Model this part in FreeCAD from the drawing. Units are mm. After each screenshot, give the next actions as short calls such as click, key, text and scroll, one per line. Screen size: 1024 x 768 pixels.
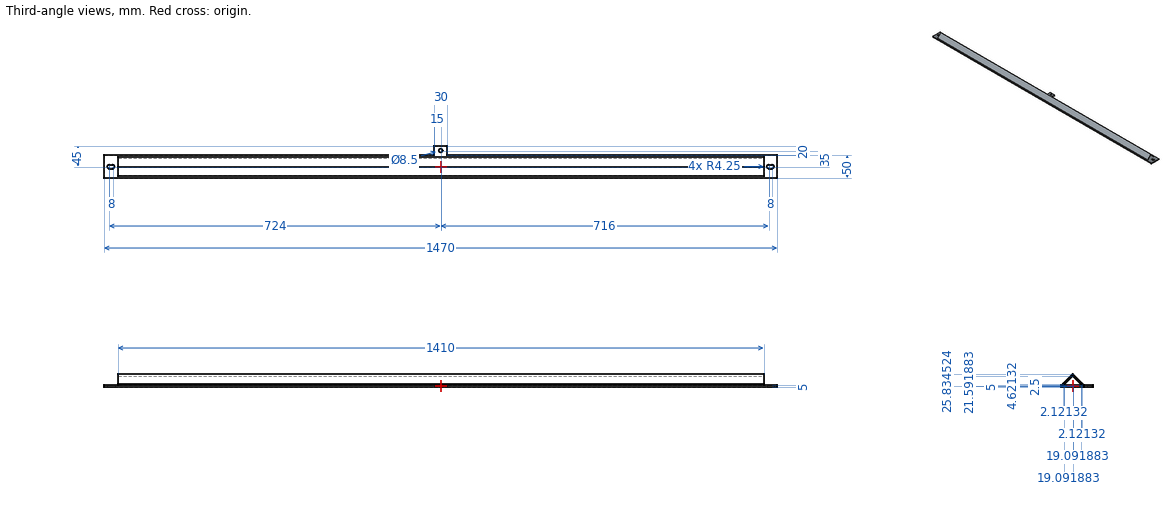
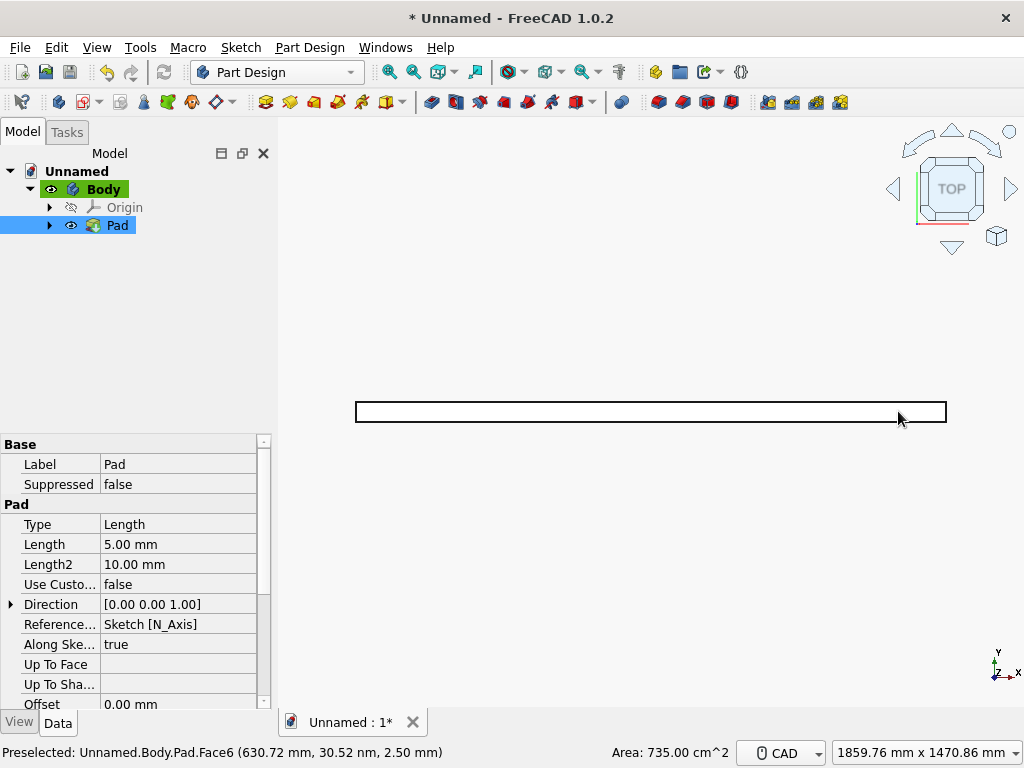
click(84, 102)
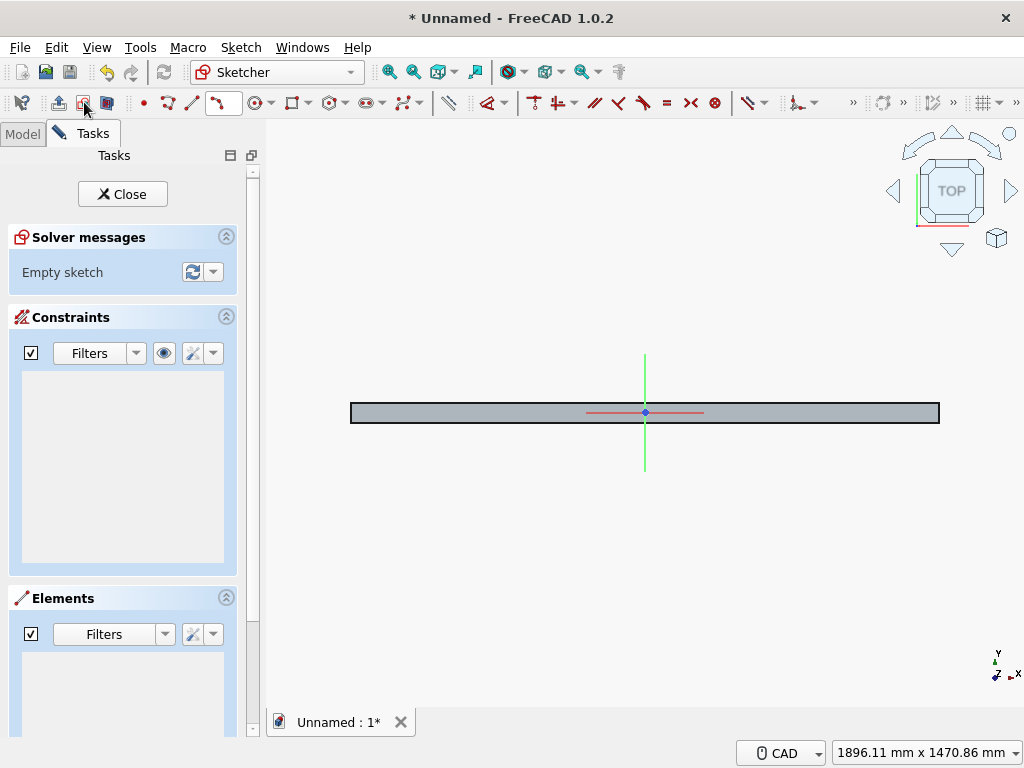
scroll(437, 413, down, 2)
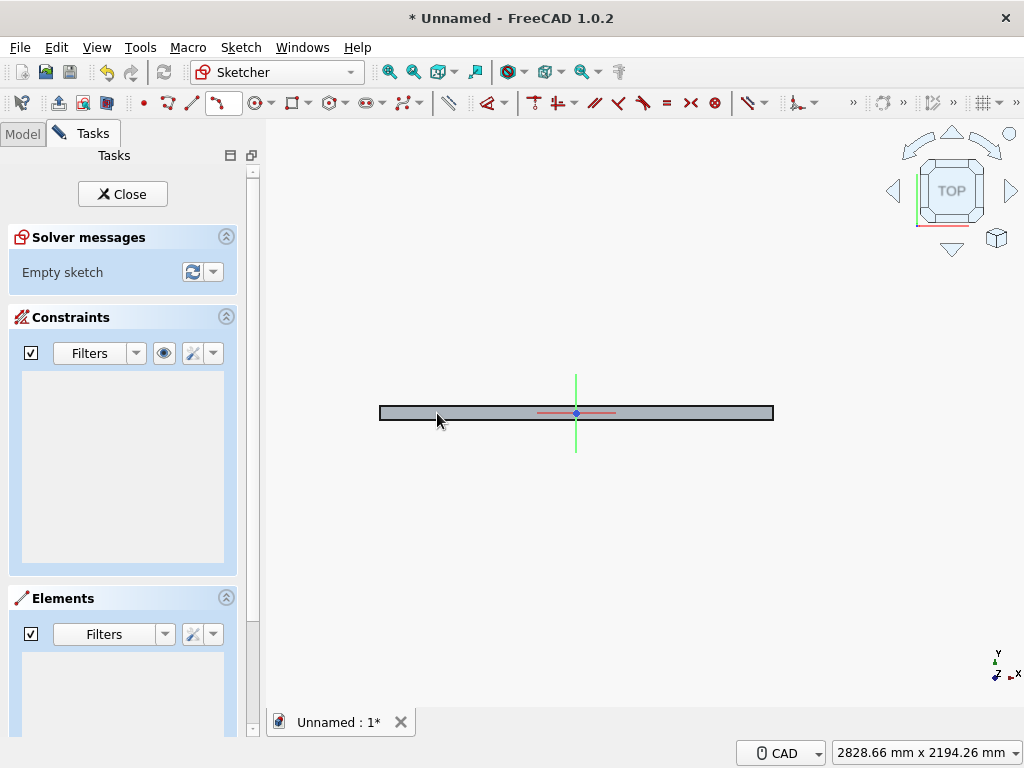
click(366, 104)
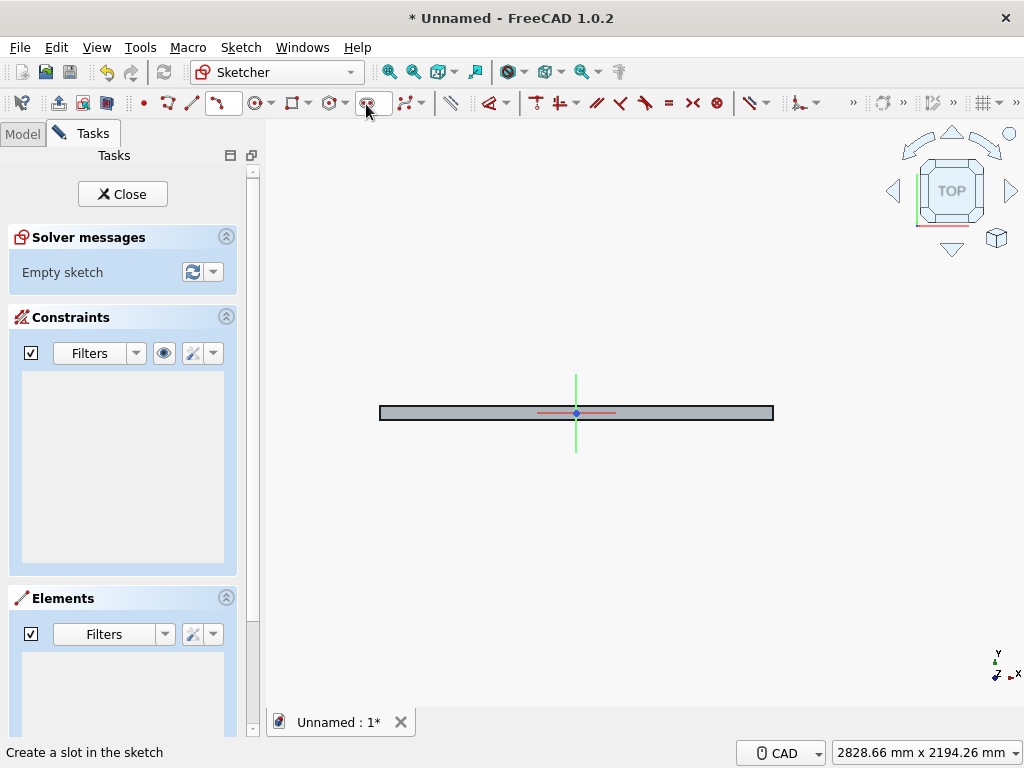
scroll(768, 413, up, 15)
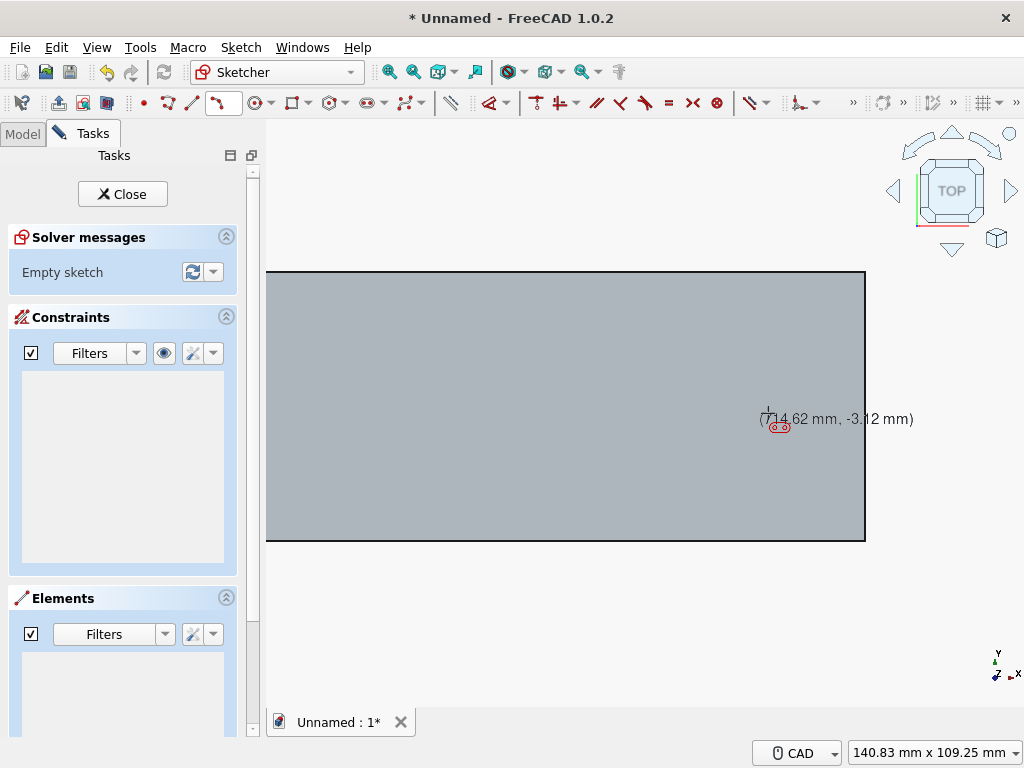
scroll(769, 413, down, 15)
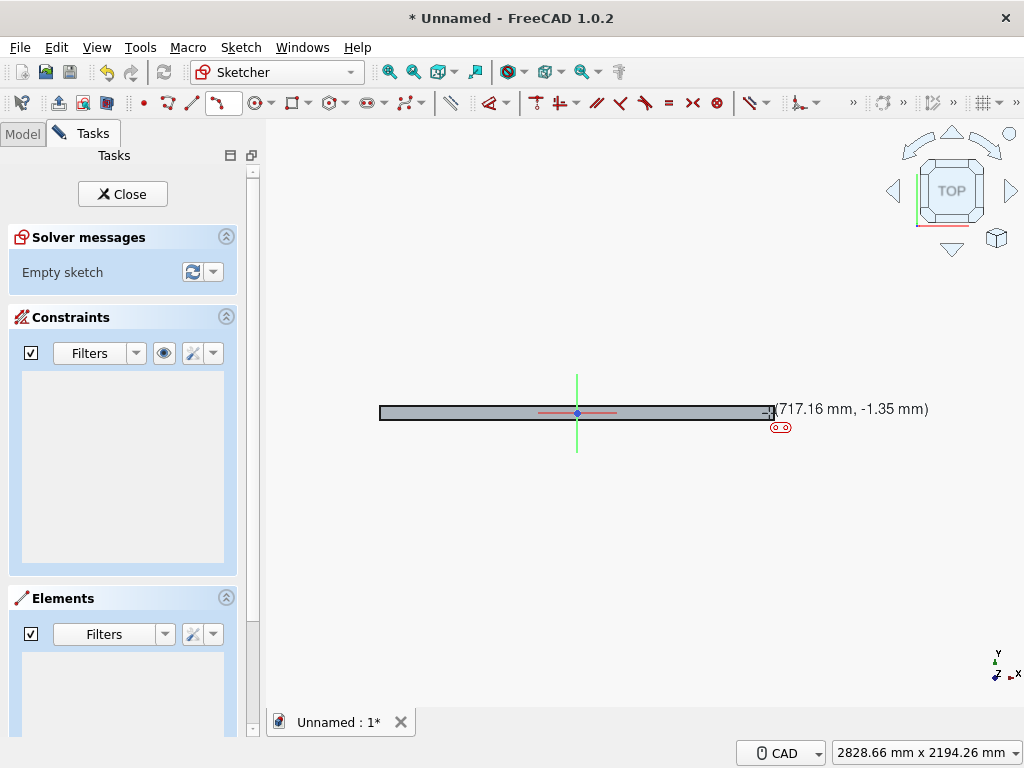
click(769, 413)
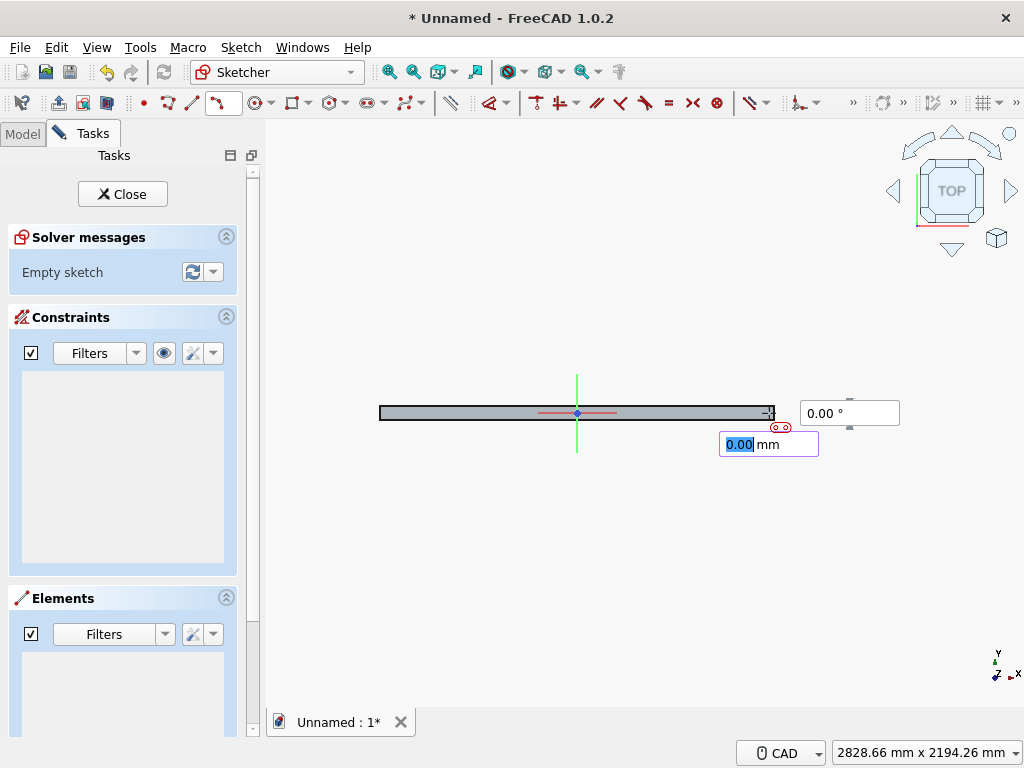
scroll(771, 413, up, 11)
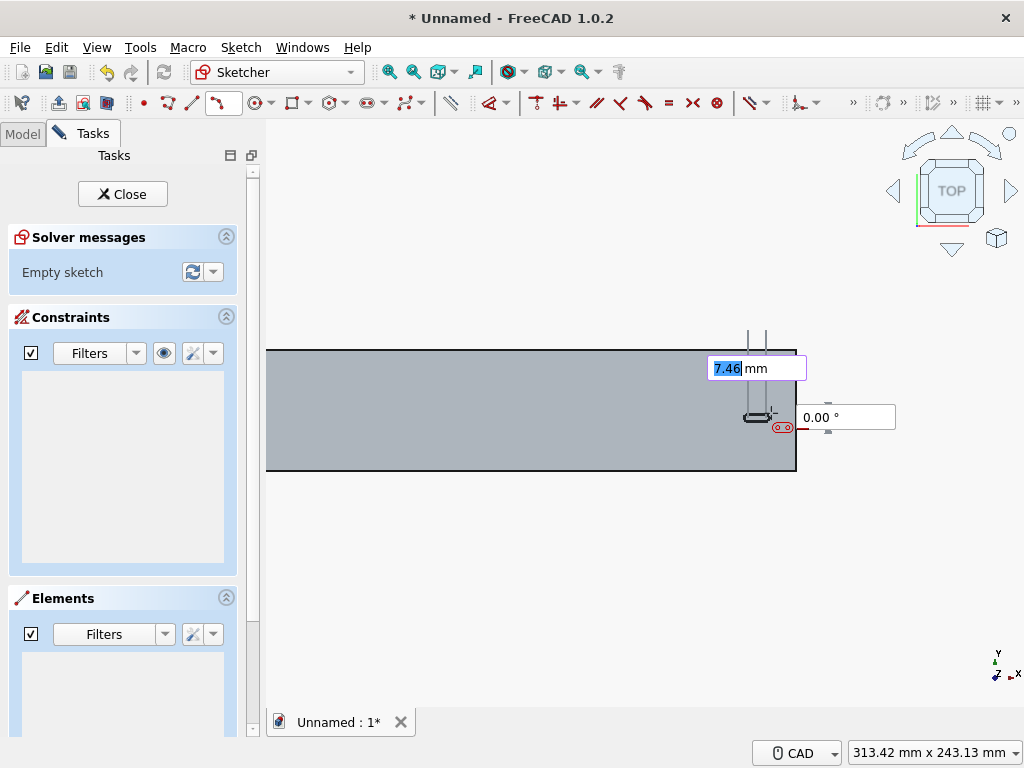
click(770, 401)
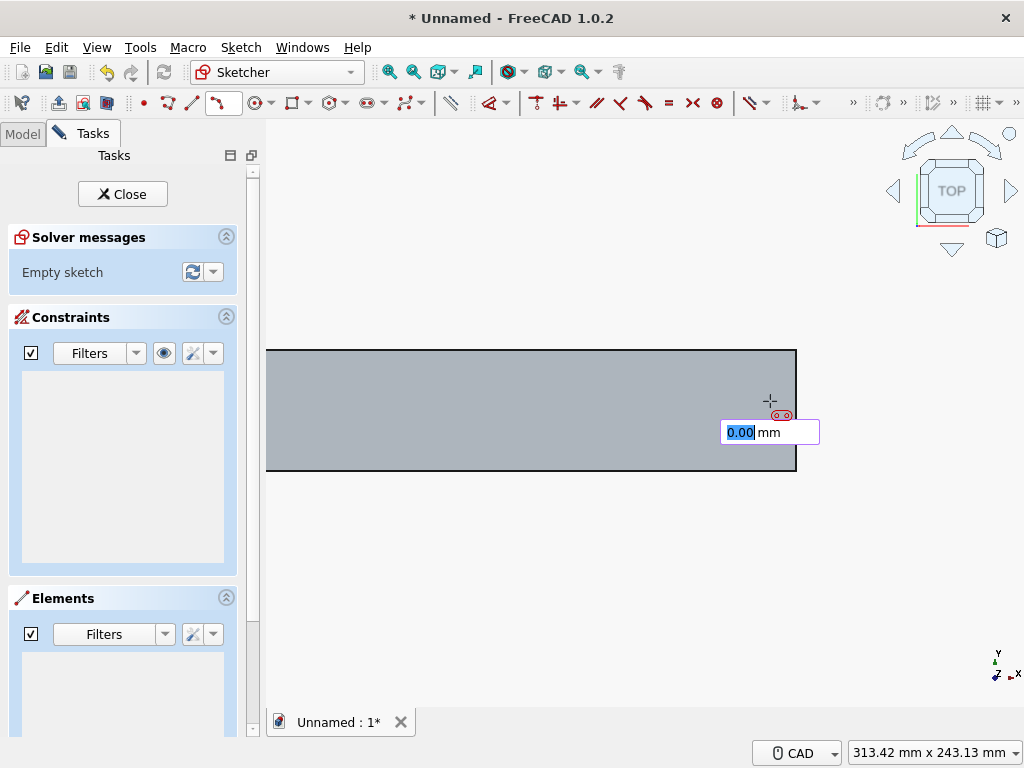
scroll(760, 400, up, 3)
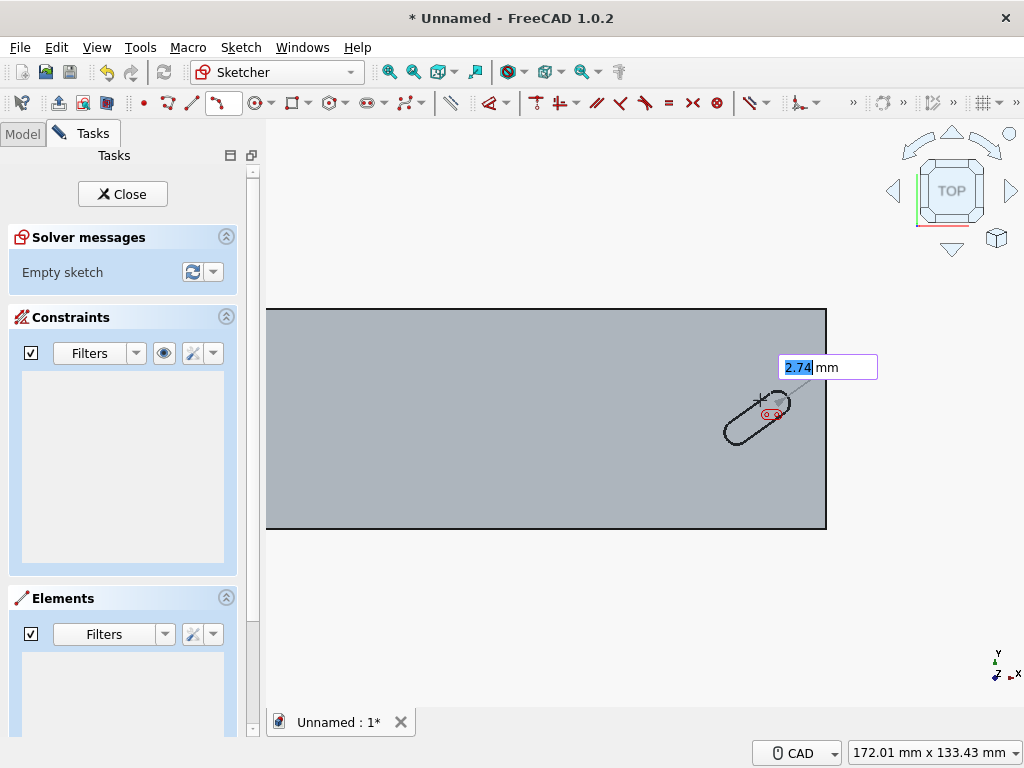
click(760, 400)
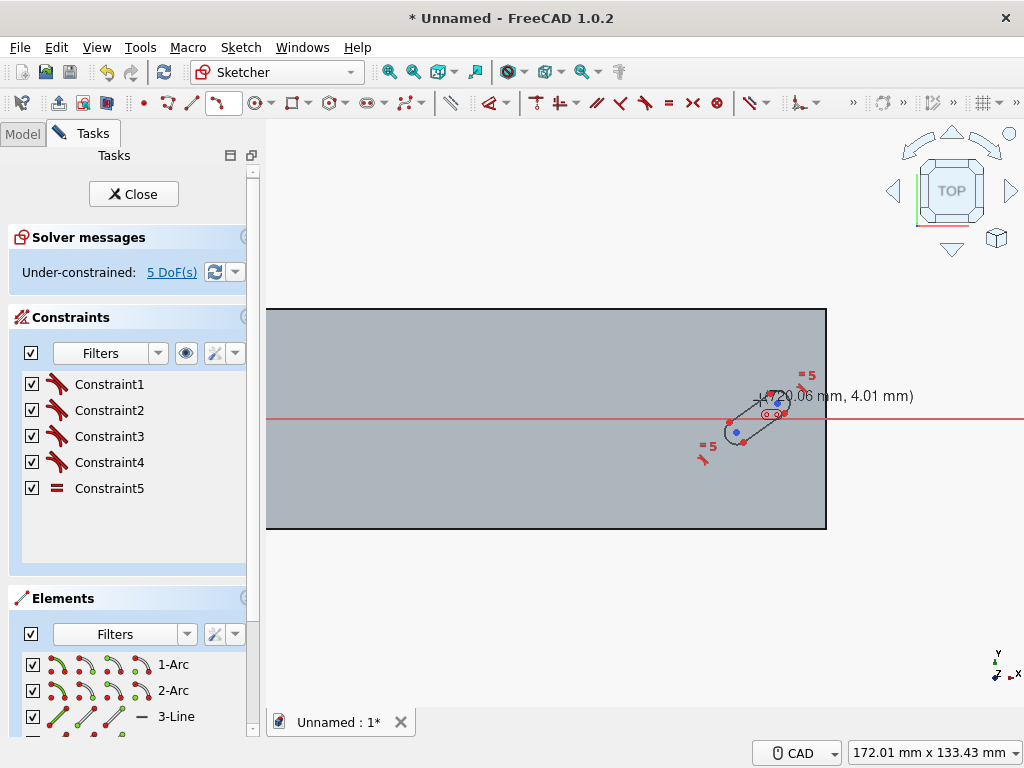
scroll(770, 413, down, 14)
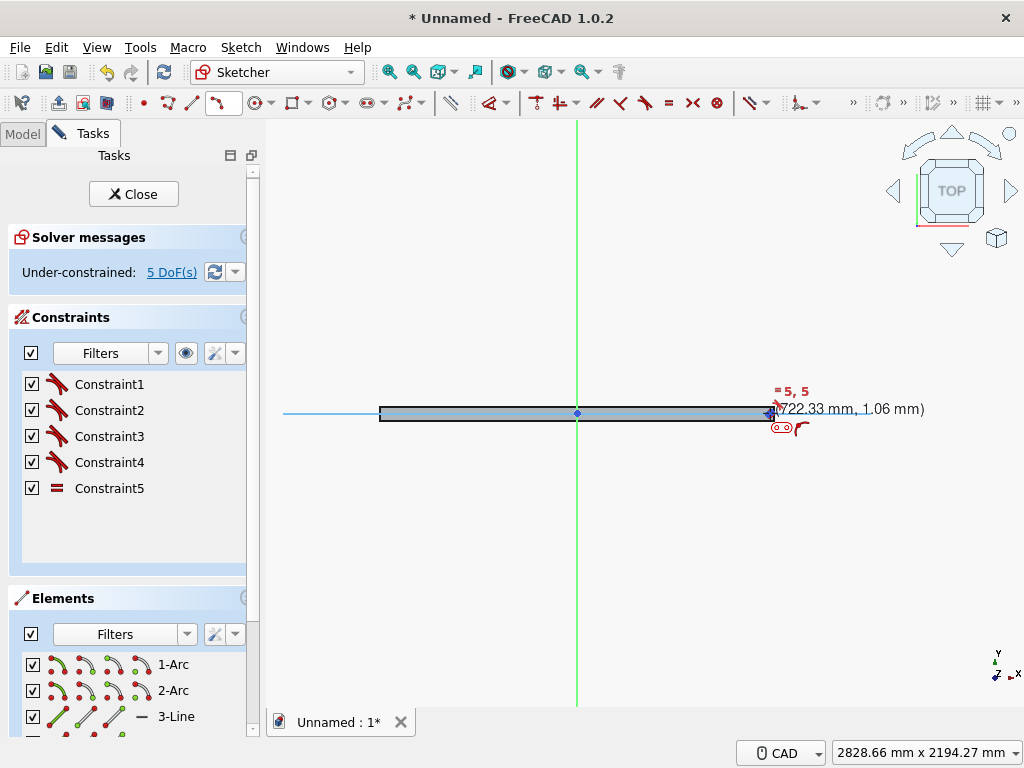
scroll(383, 414, up, 15)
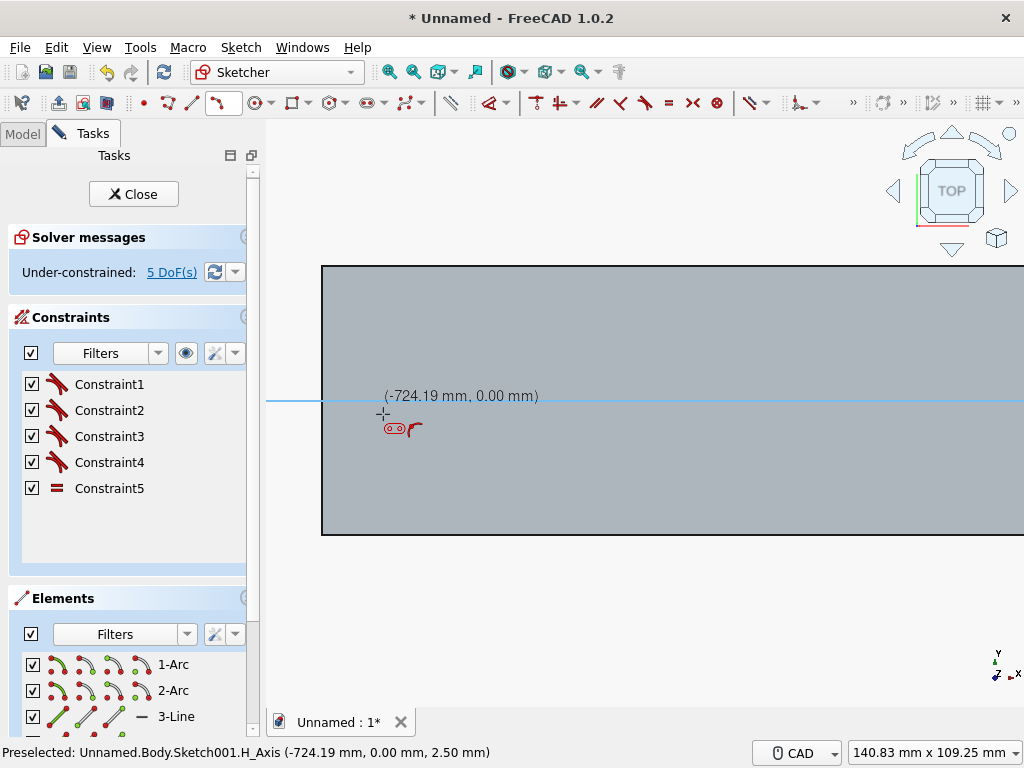
scroll(383, 414, down, 15)